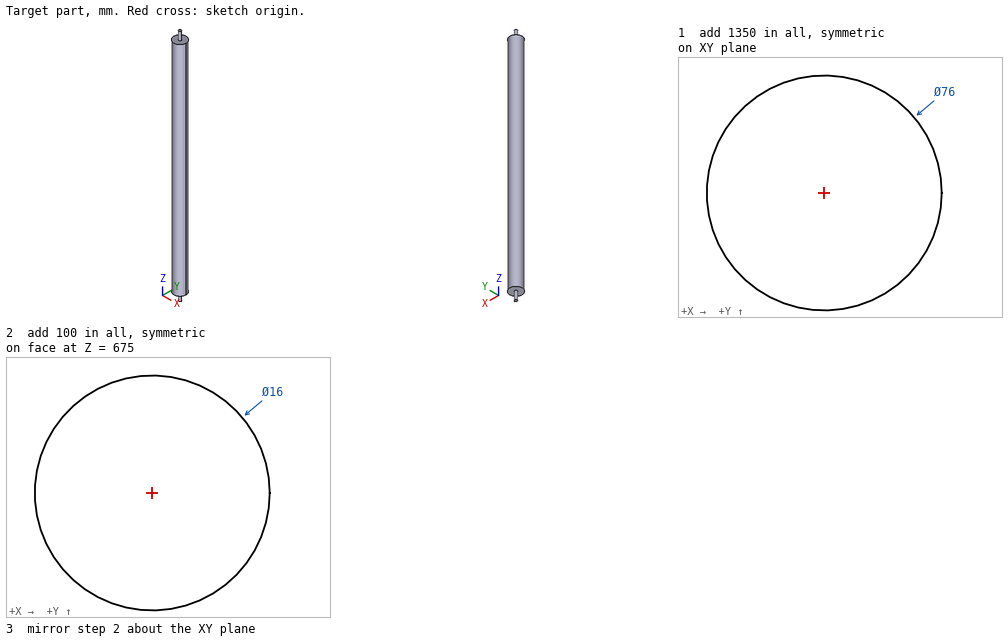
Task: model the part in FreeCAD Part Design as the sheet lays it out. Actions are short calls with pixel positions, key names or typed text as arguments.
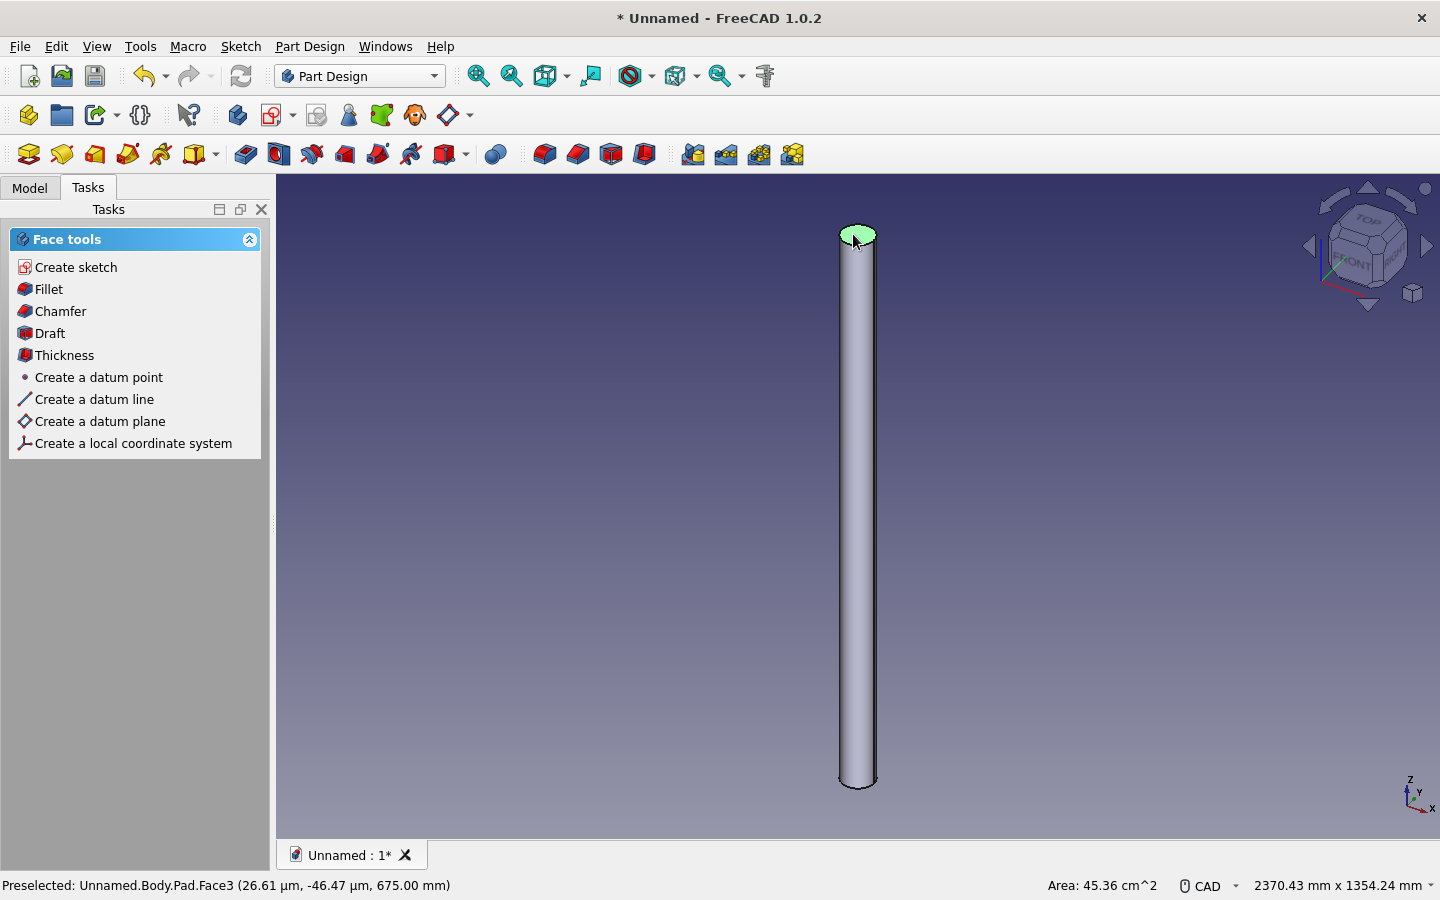
click(270, 116)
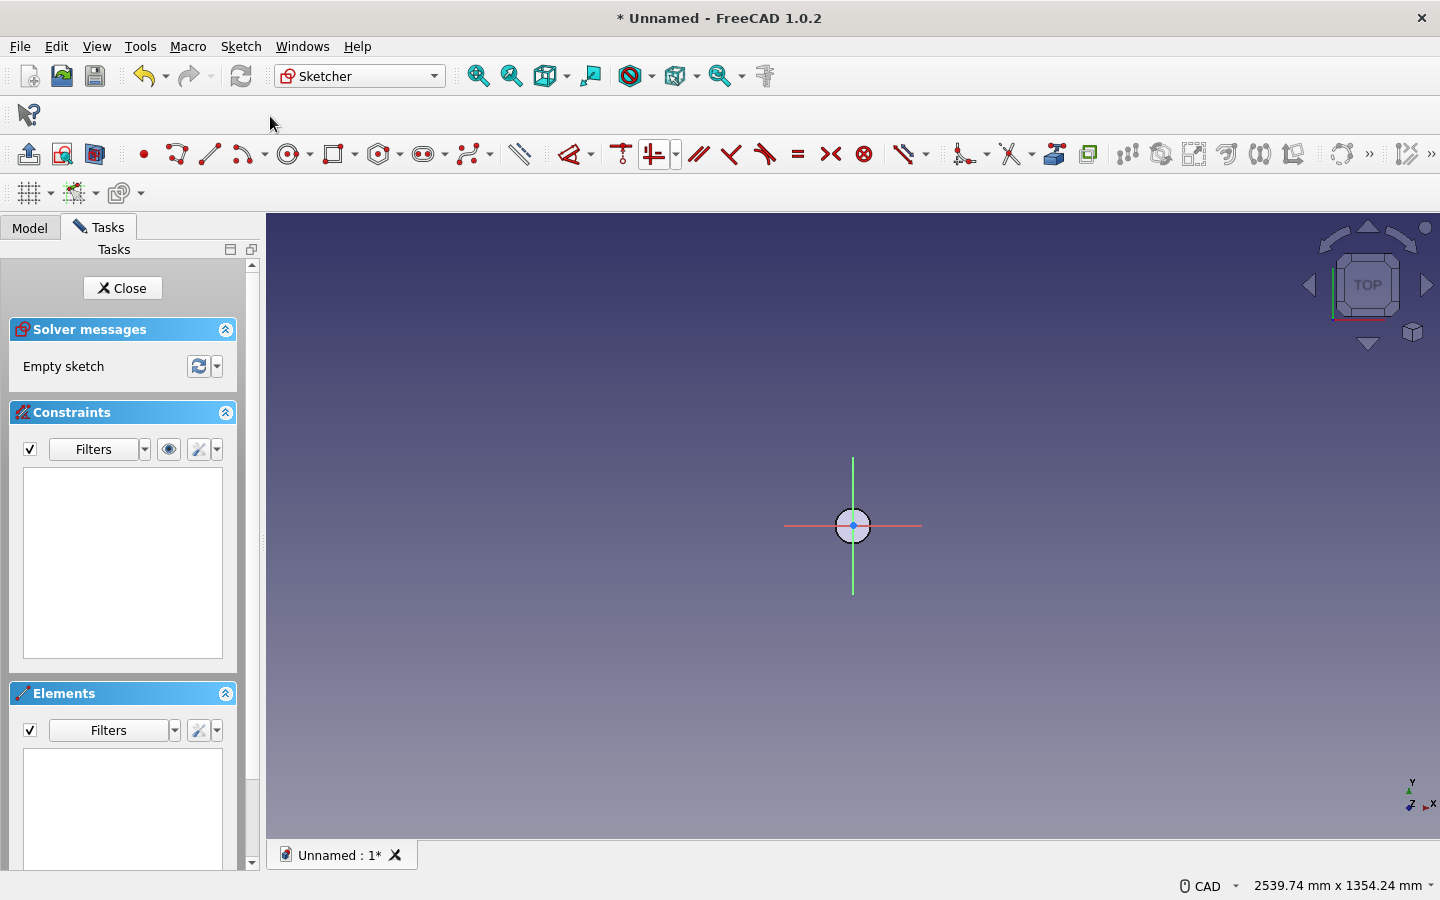
scroll(857, 526, up, 15)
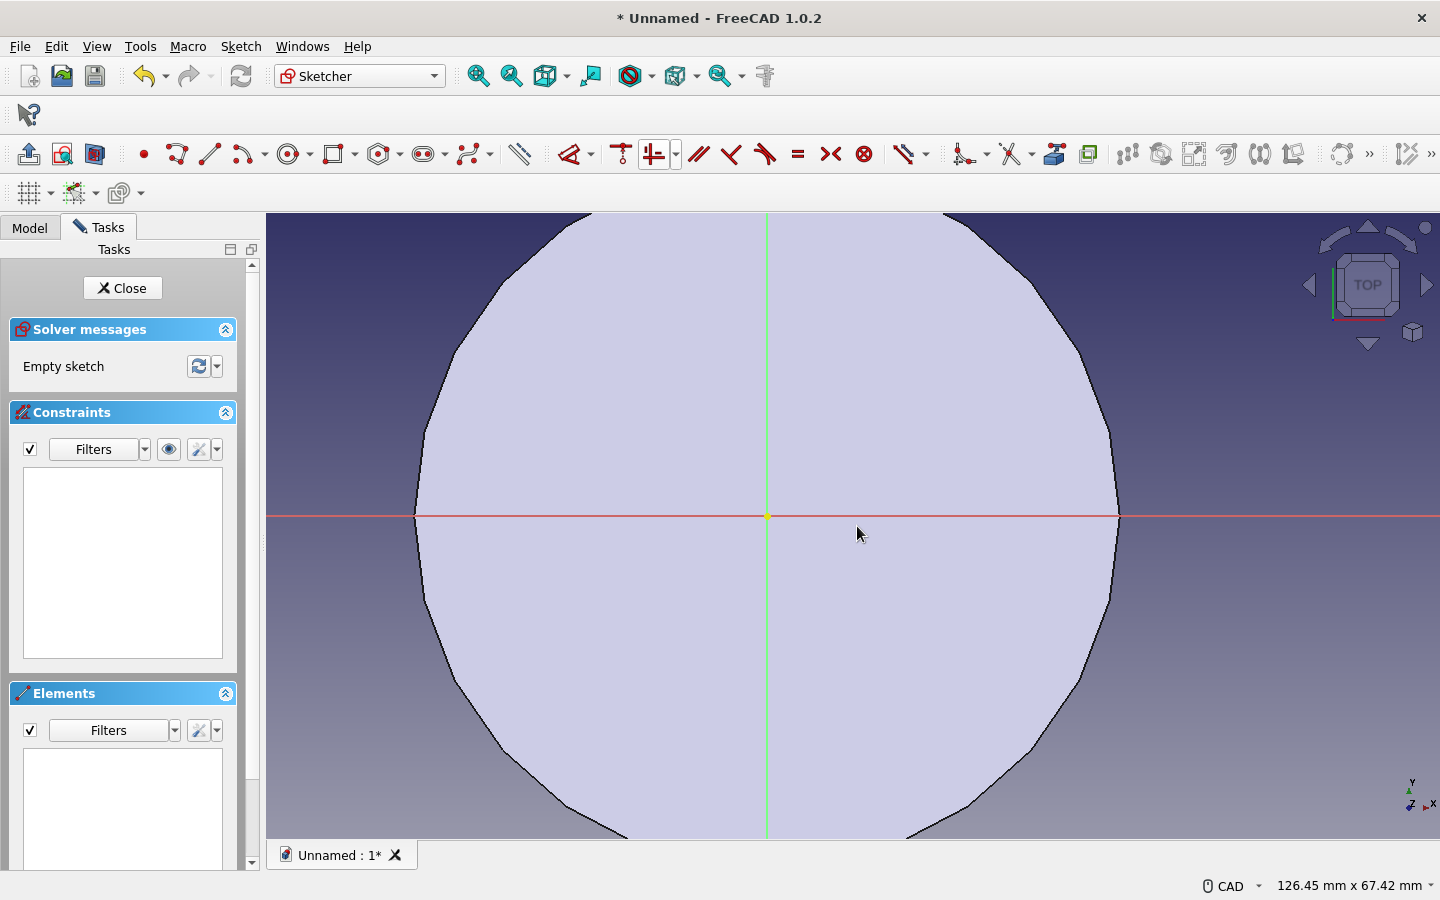
scroll(757, 511, up, 5)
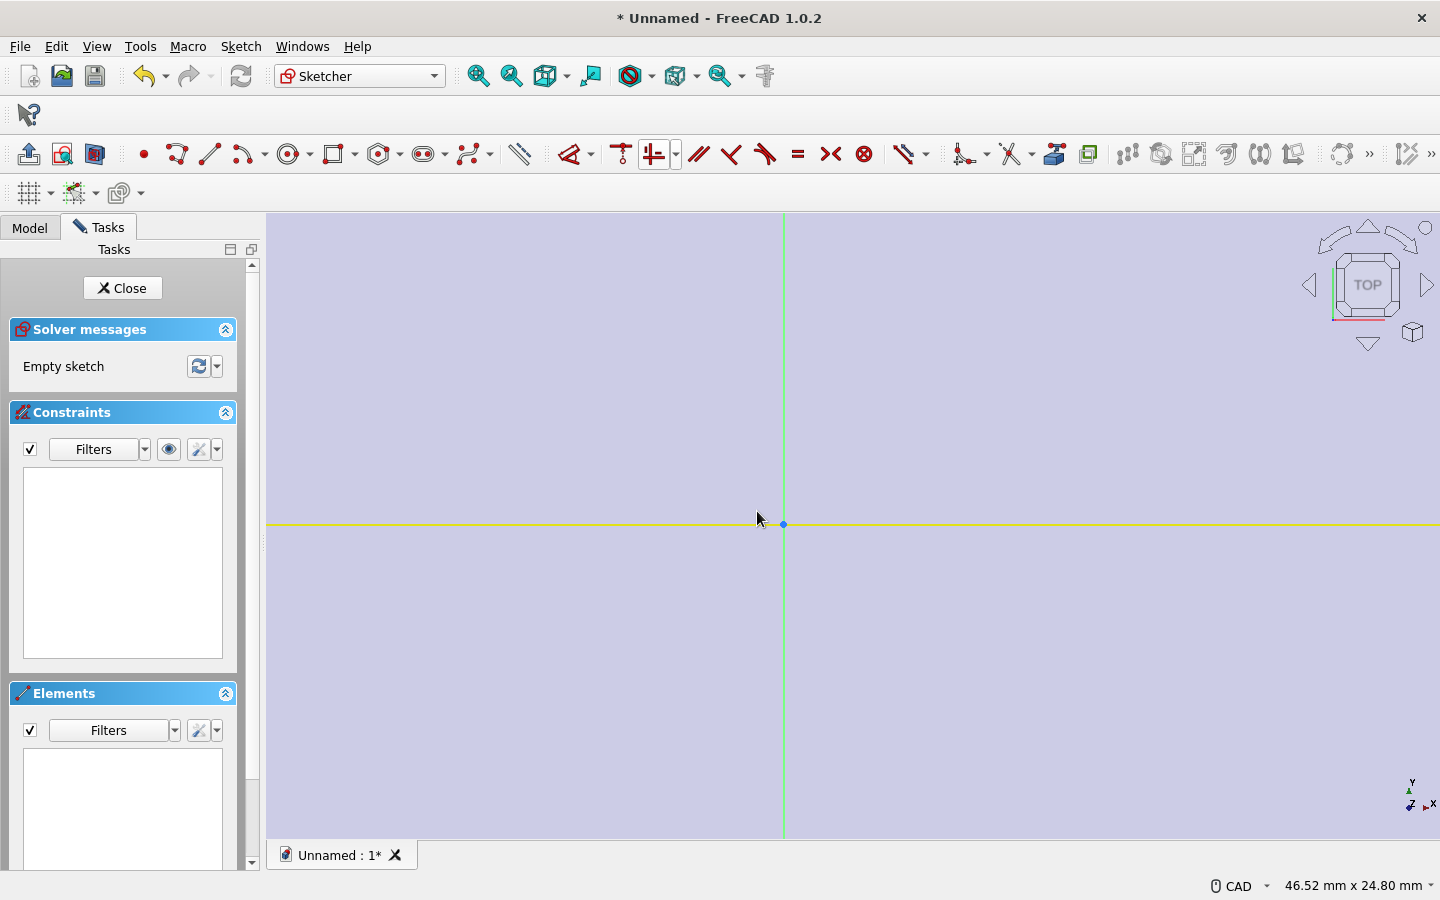
click(288, 154)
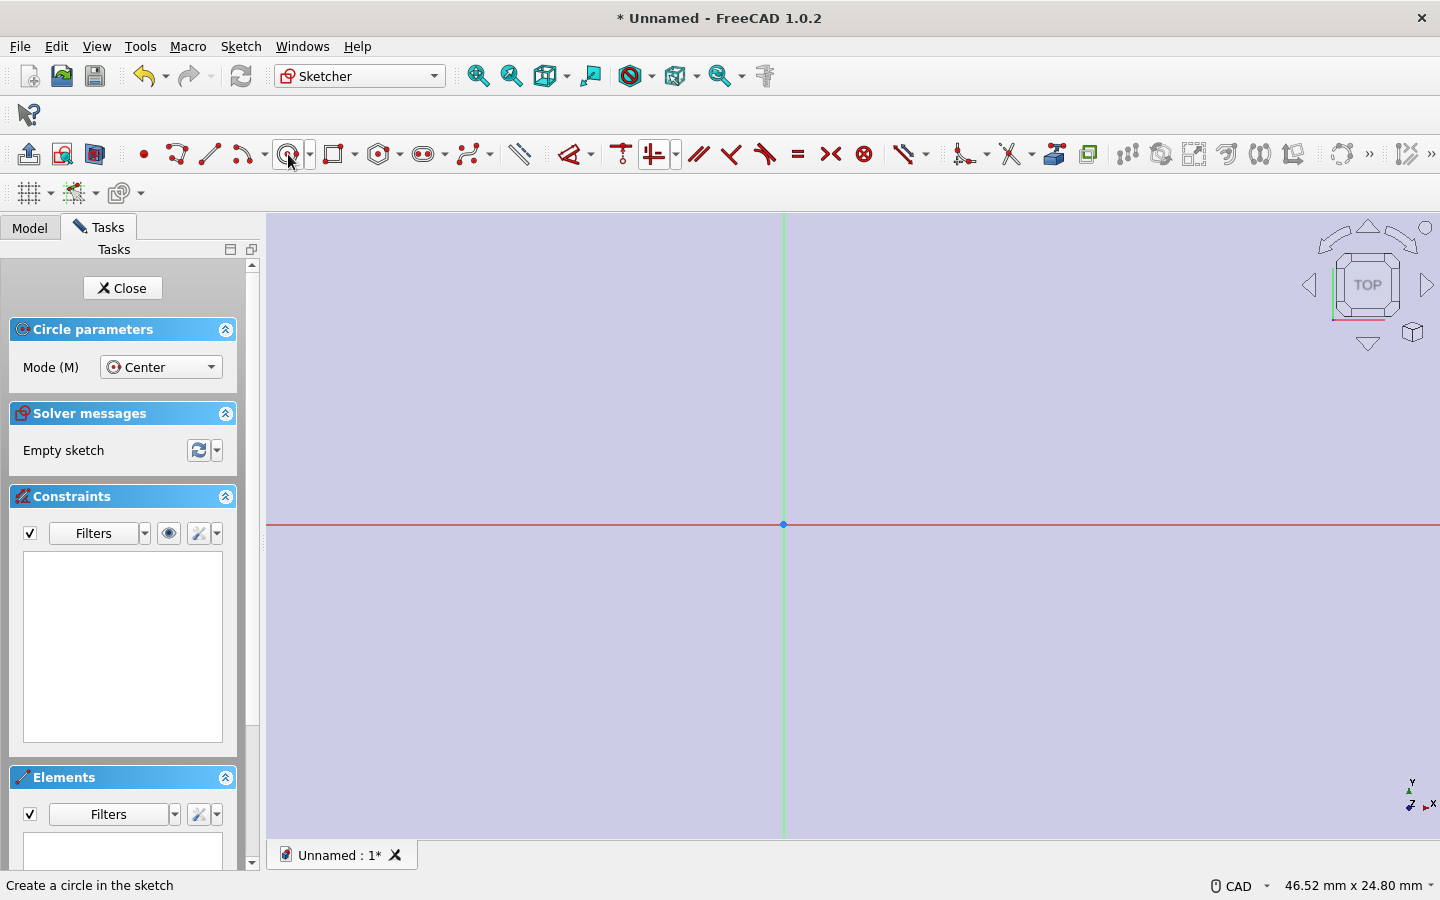
click(784, 525)
click(926, 382)
key(Escape)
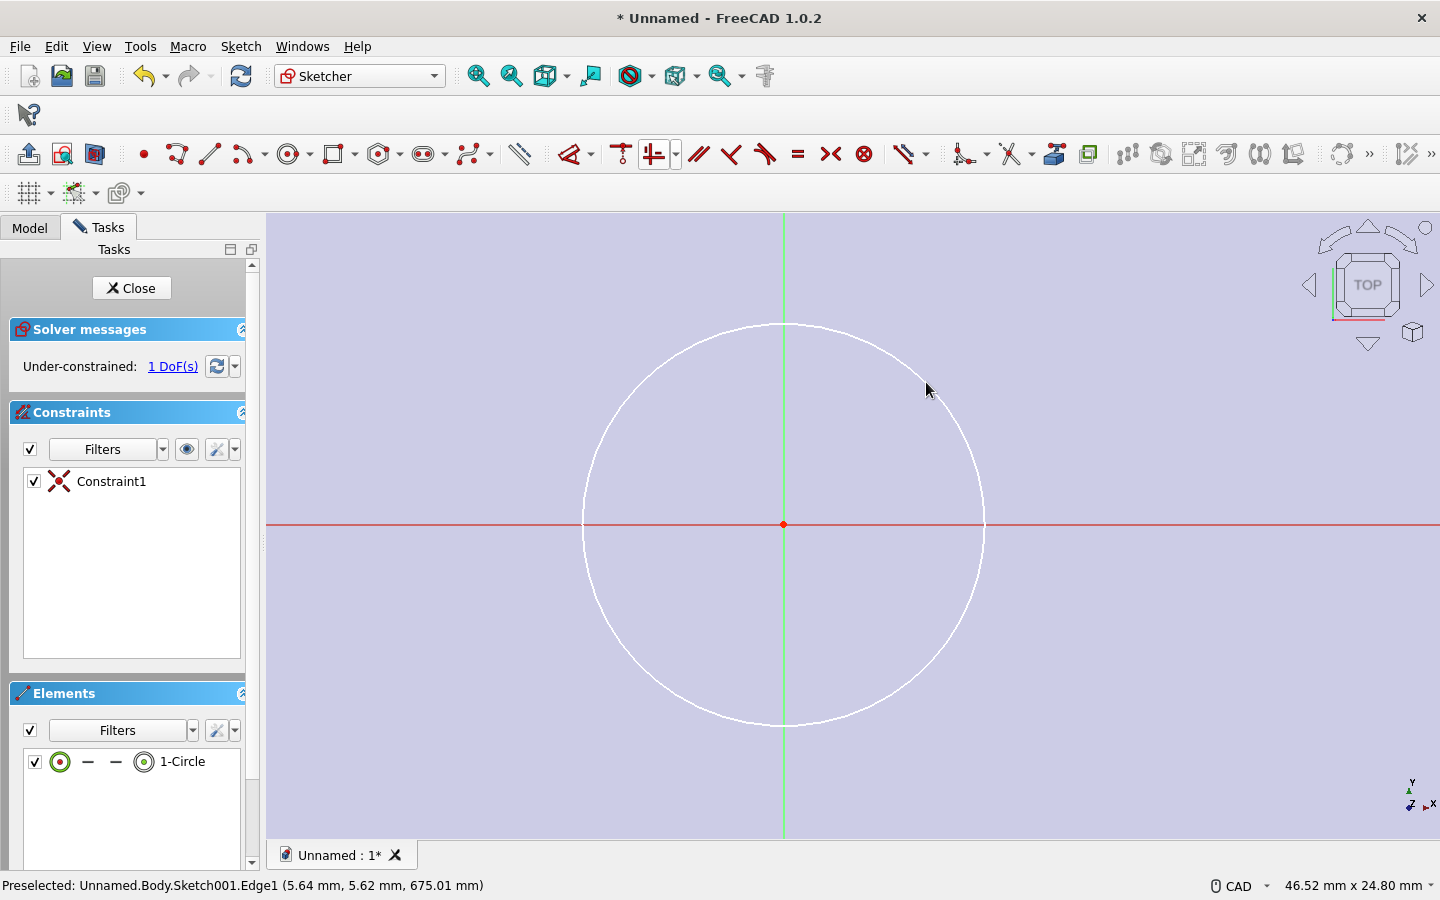
click(568, 154)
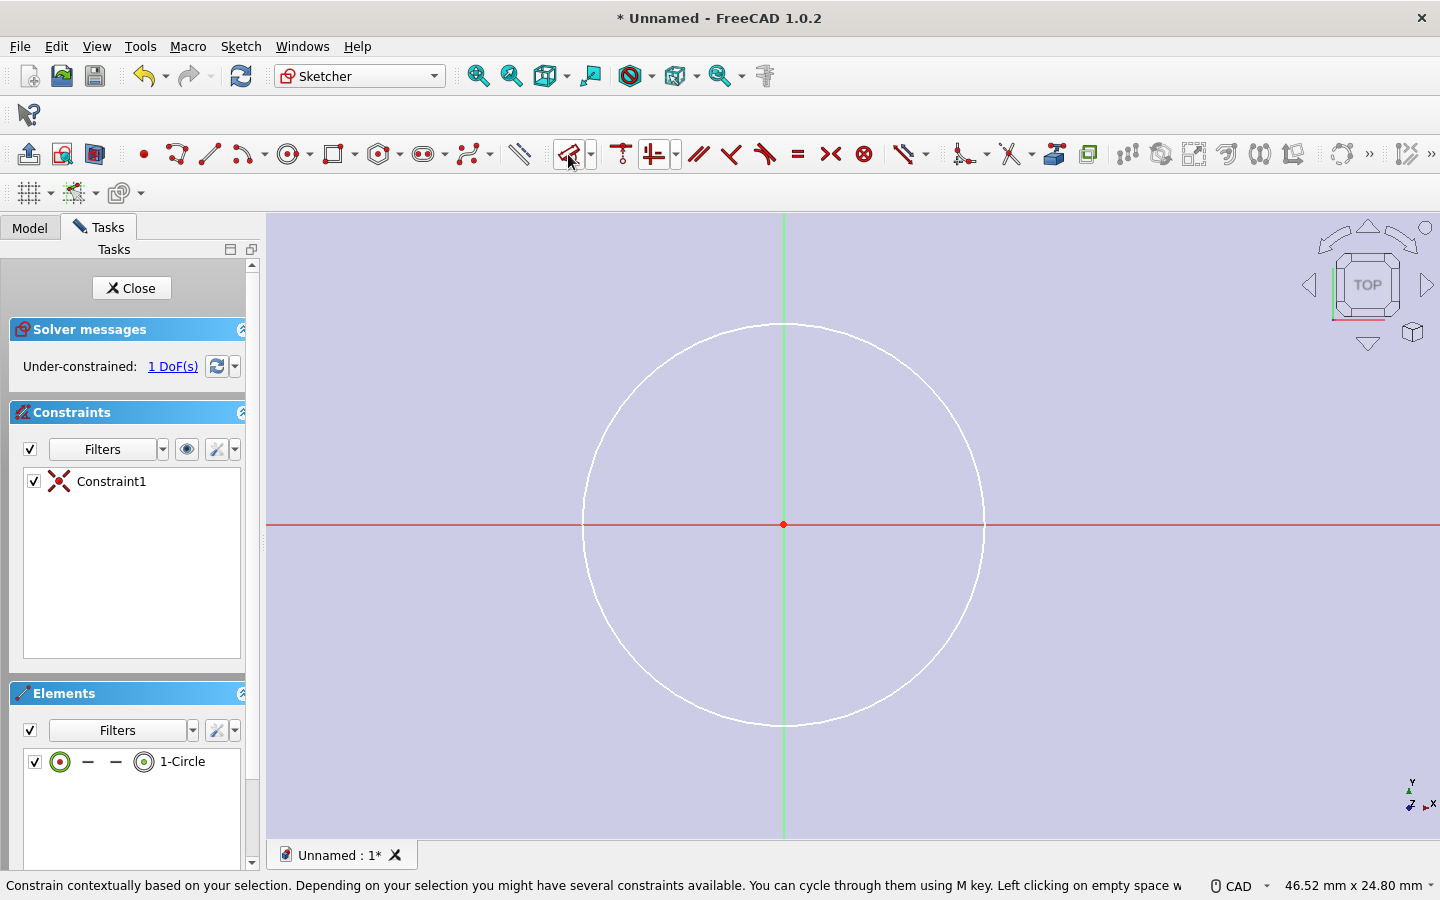
click(925, 382)
click(948, 359)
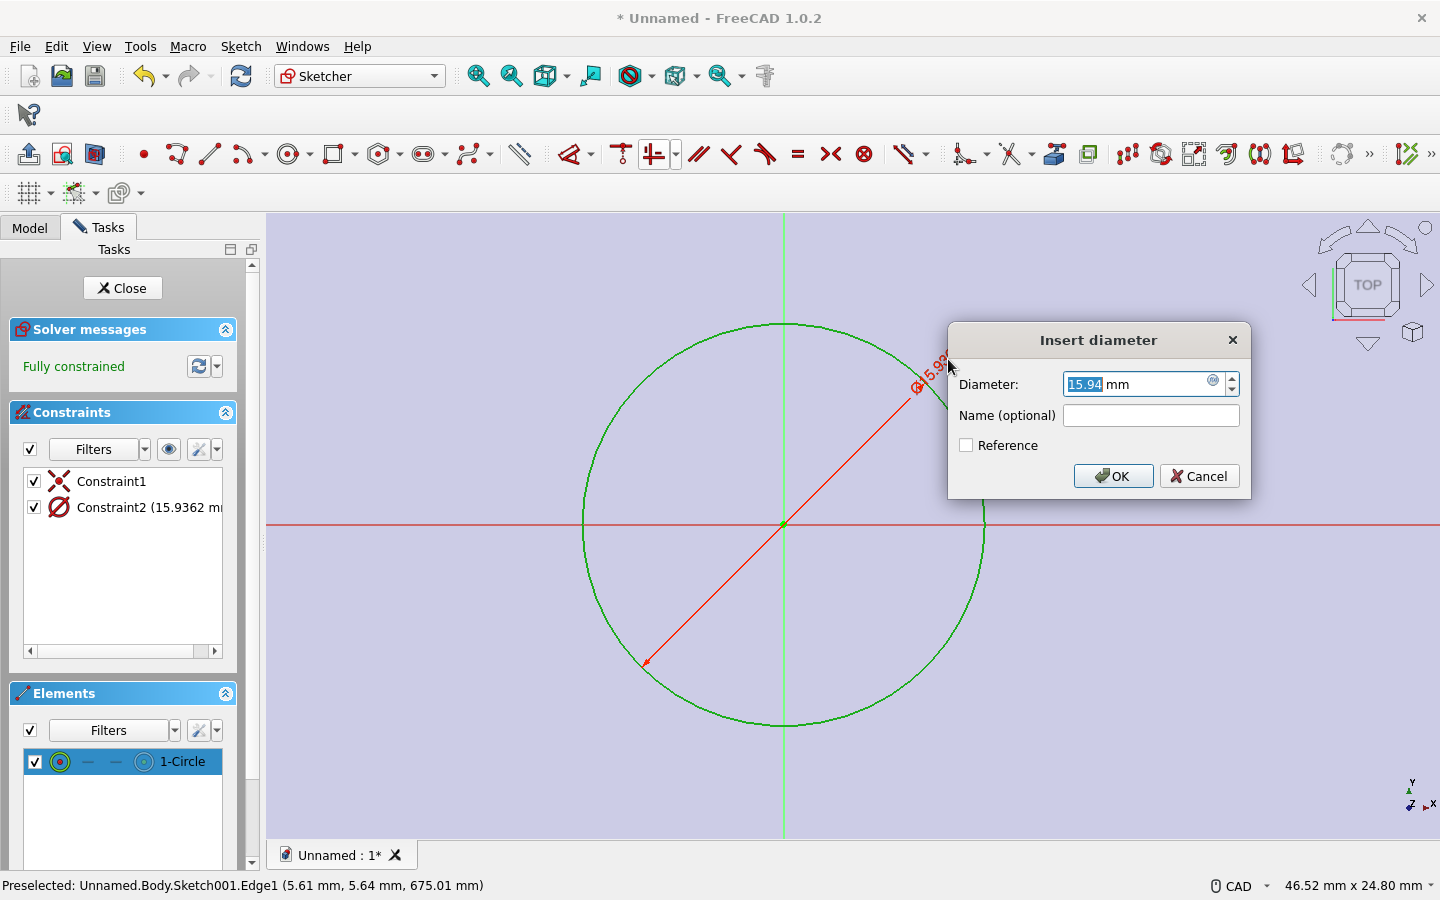
text(16)
key(Return)
key(Escape)